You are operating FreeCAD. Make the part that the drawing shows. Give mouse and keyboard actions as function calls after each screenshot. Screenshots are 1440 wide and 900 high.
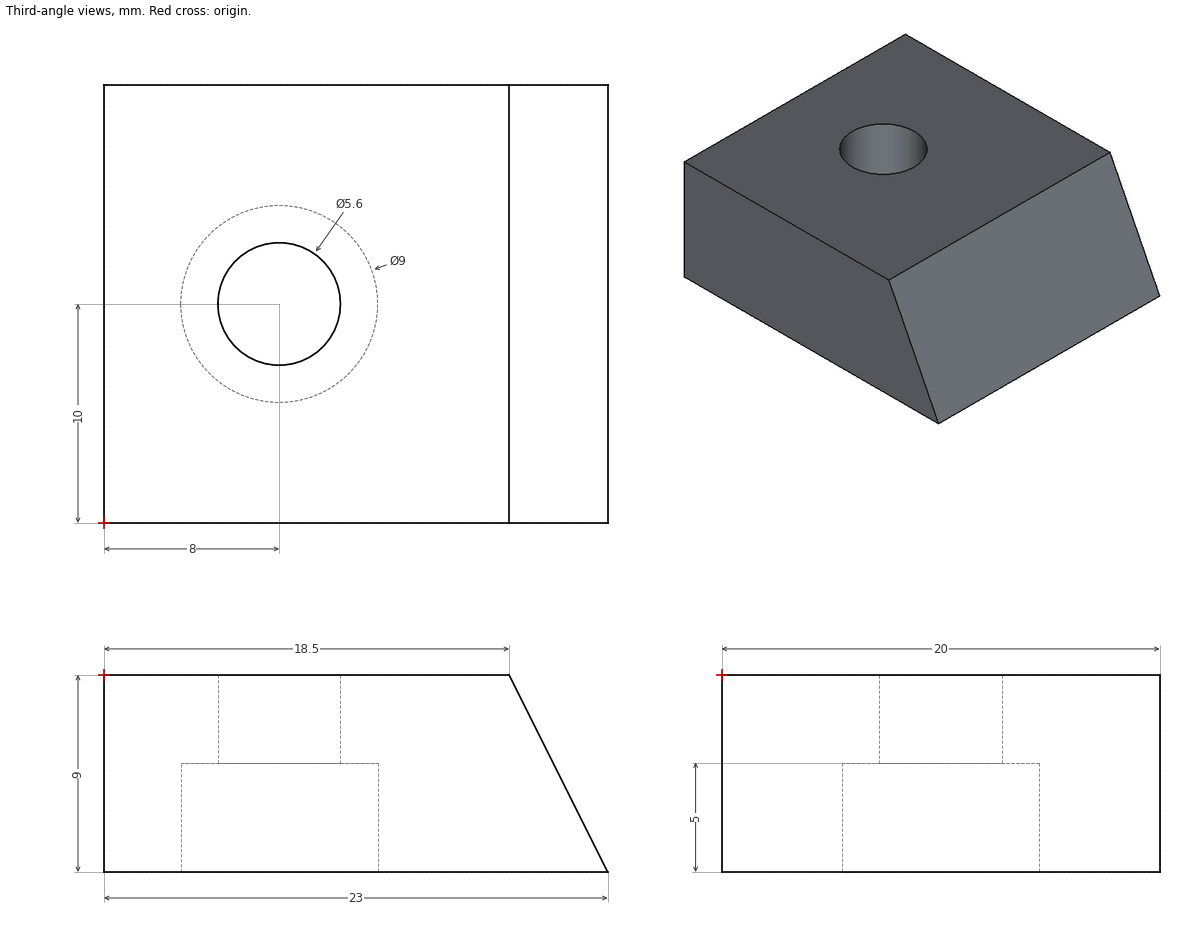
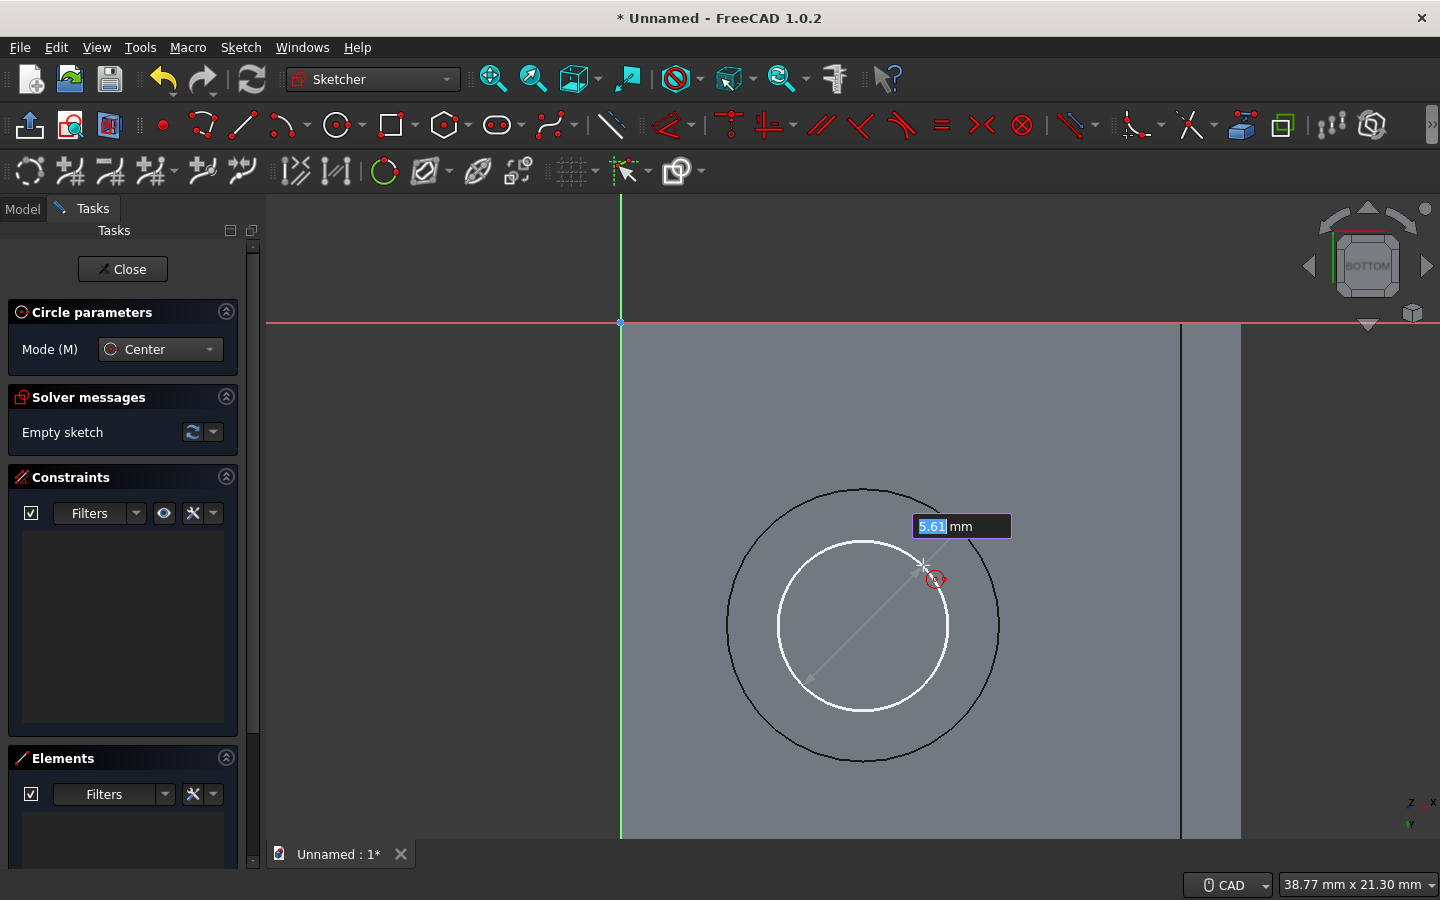
text(5.6)
key(Return)
key(Escape)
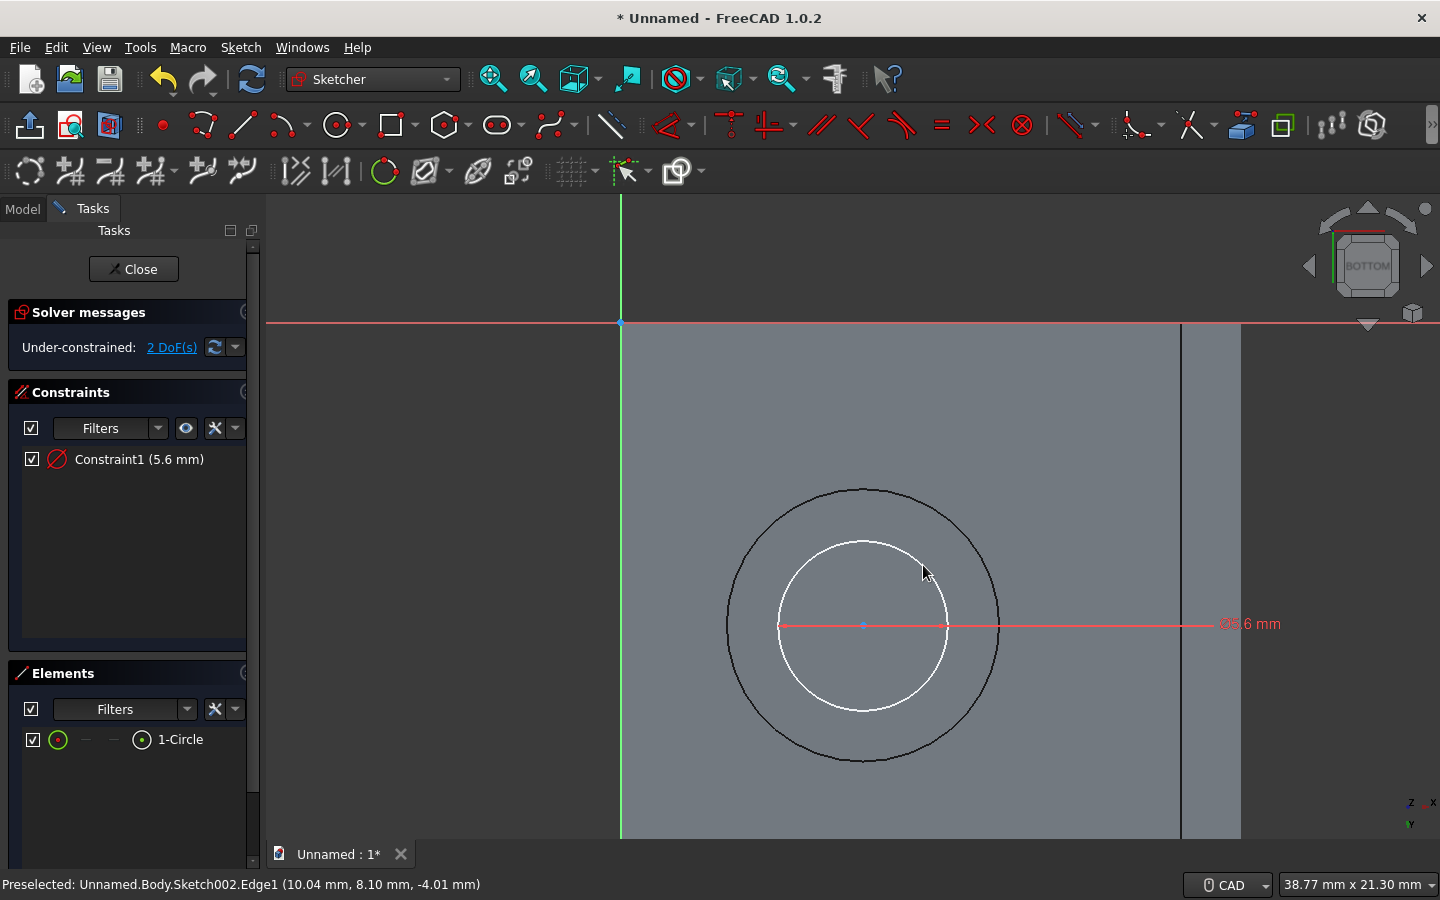
key(d)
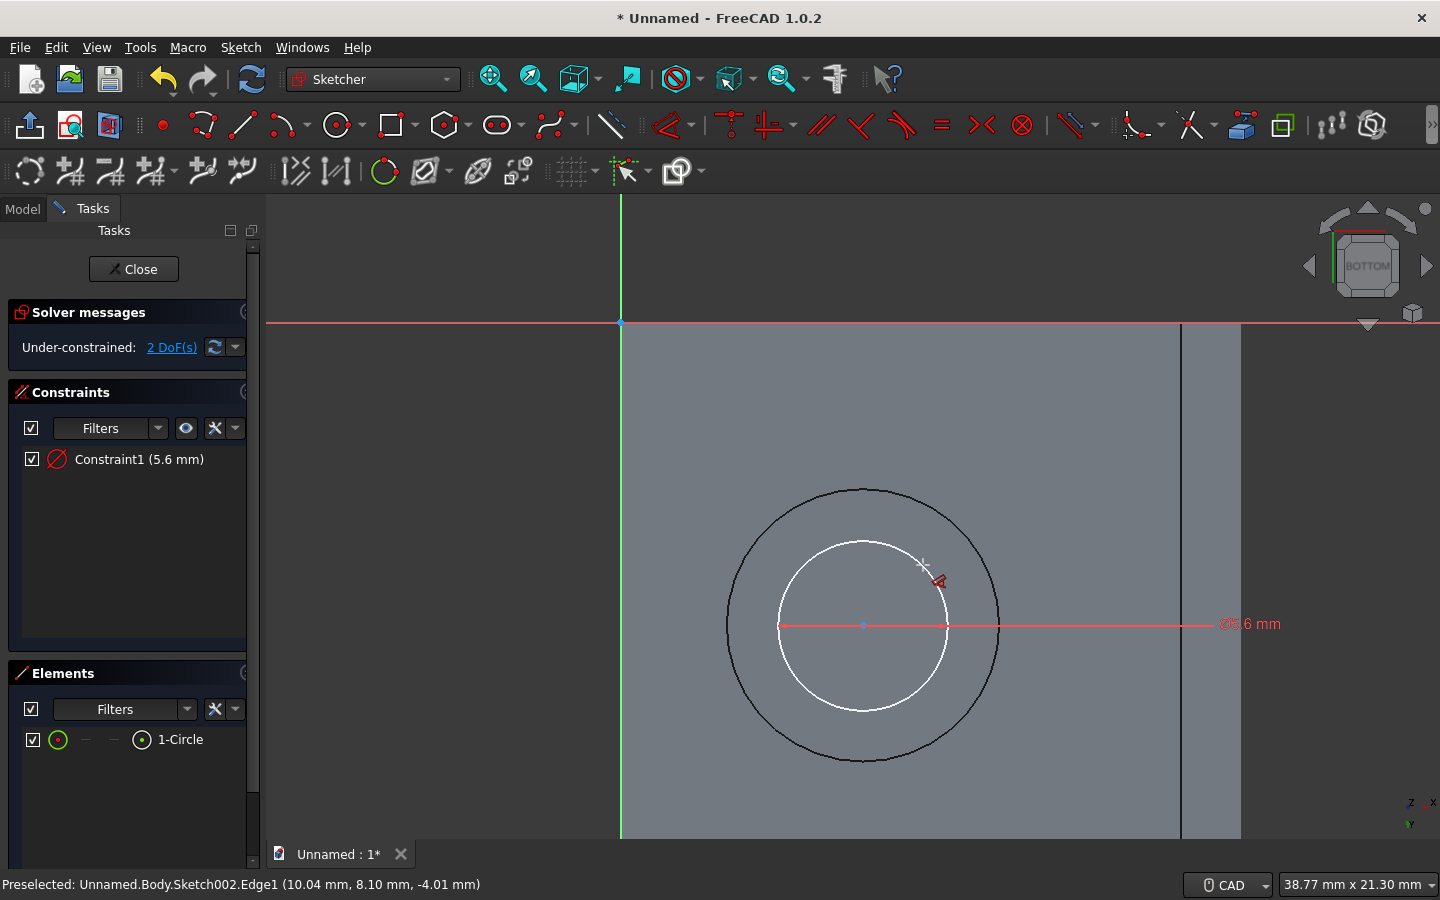
click(863, 626)
click(742, 289)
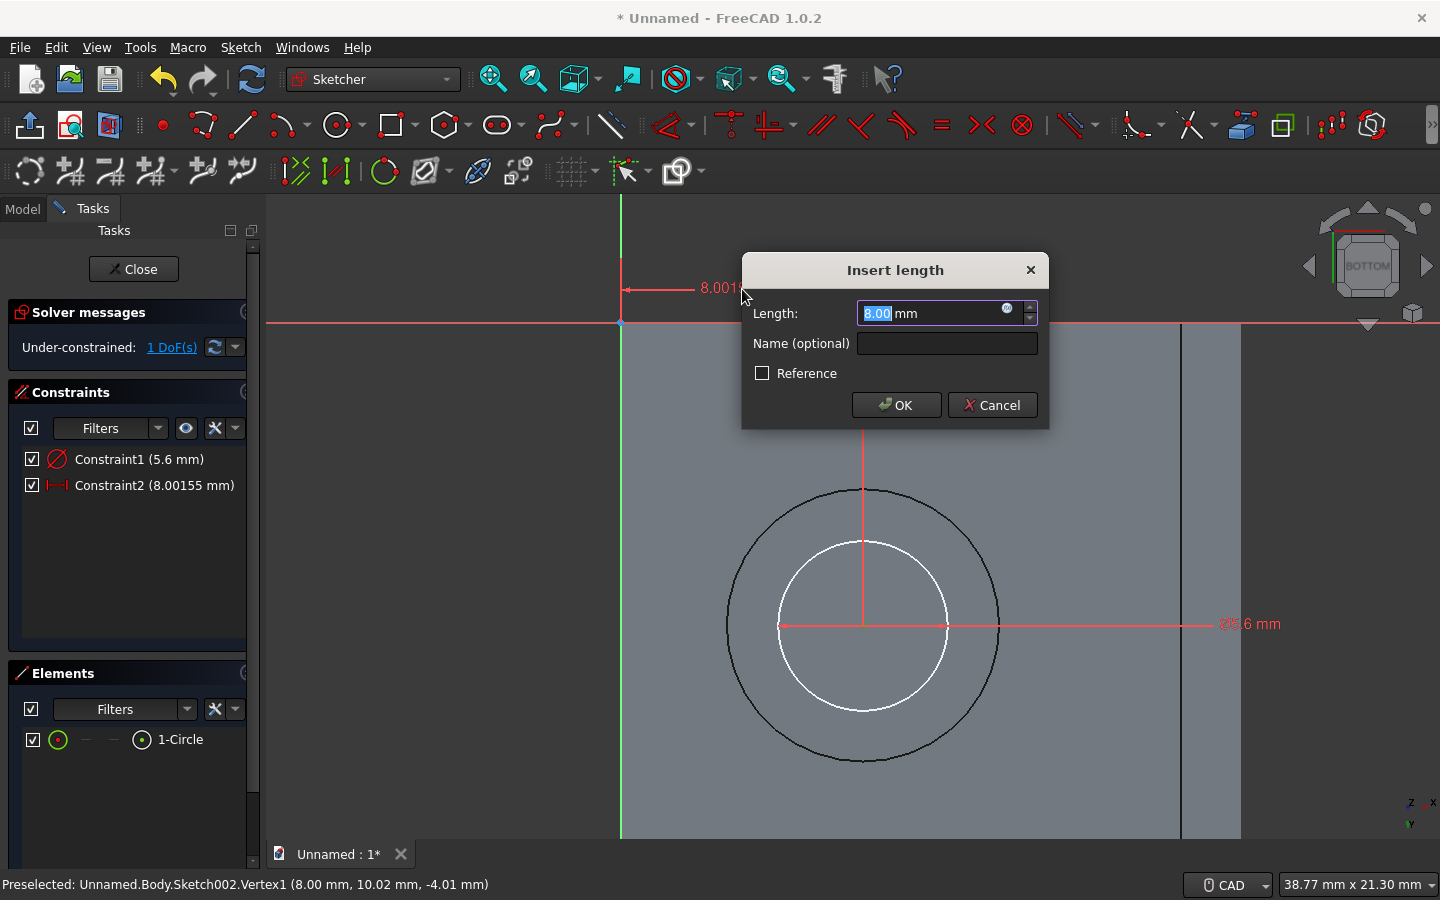
text(8)
key(Return)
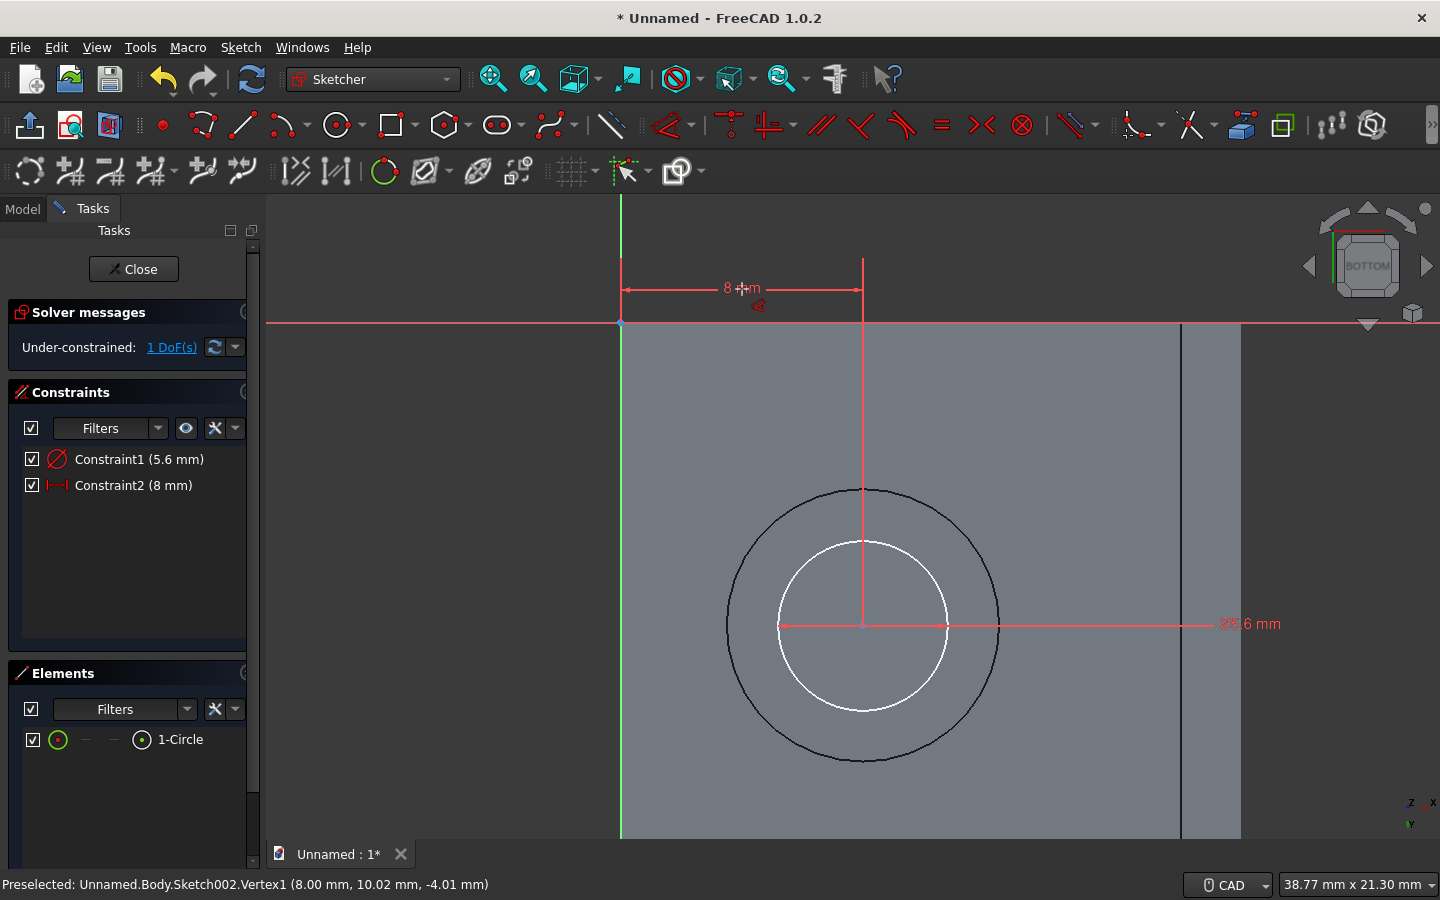
click(863, 626)
click(587, 474)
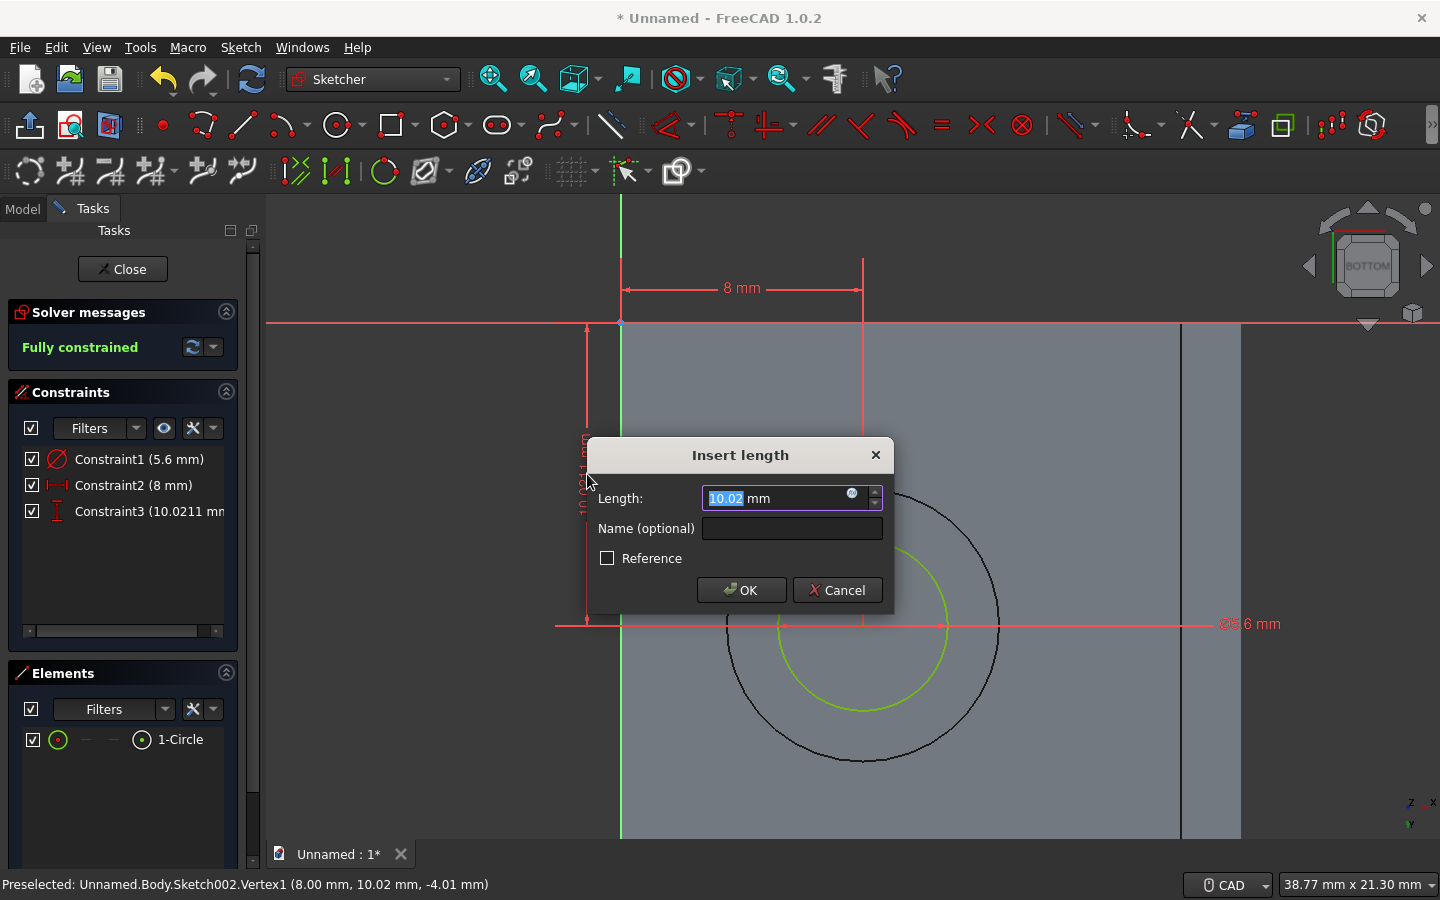
text(10)
key(Return)
key(Escape)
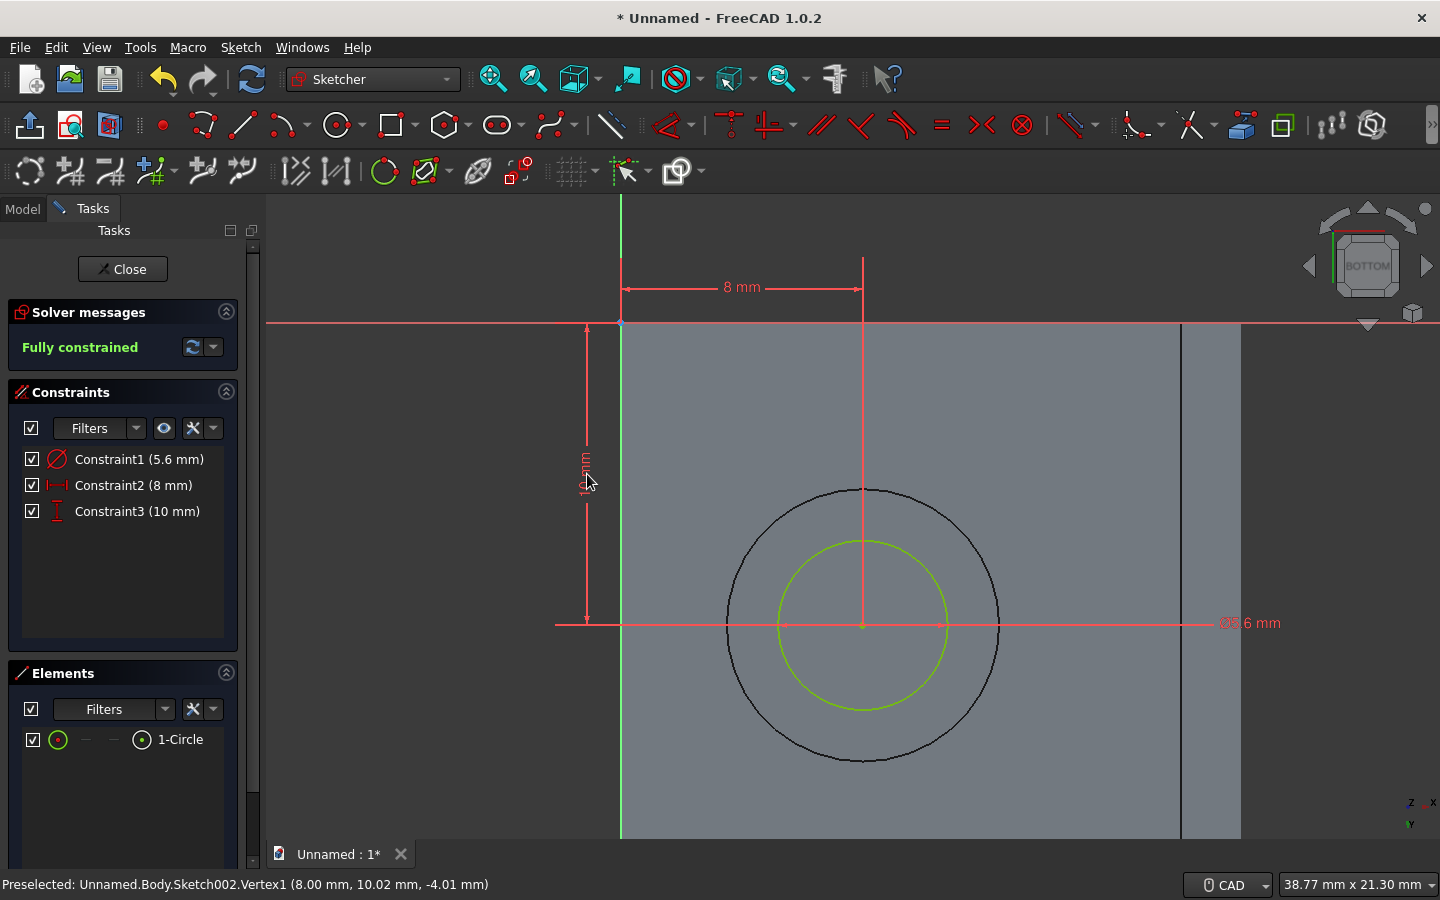
click(123, 269)